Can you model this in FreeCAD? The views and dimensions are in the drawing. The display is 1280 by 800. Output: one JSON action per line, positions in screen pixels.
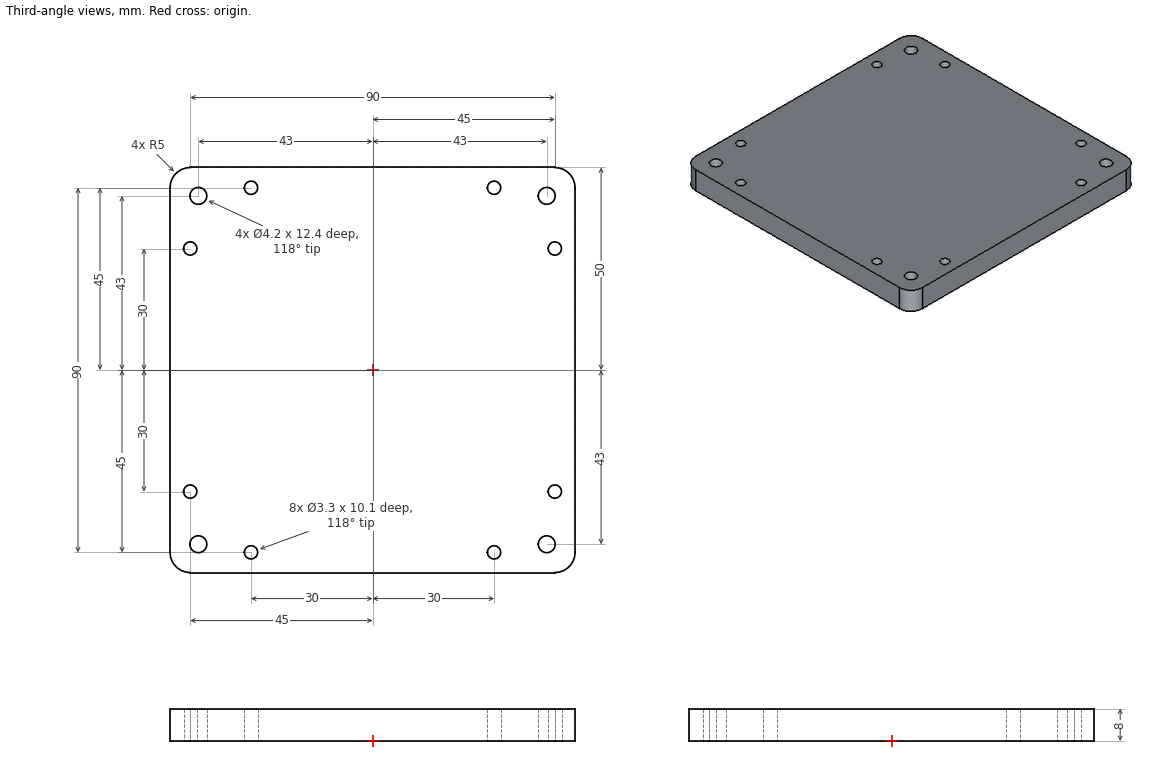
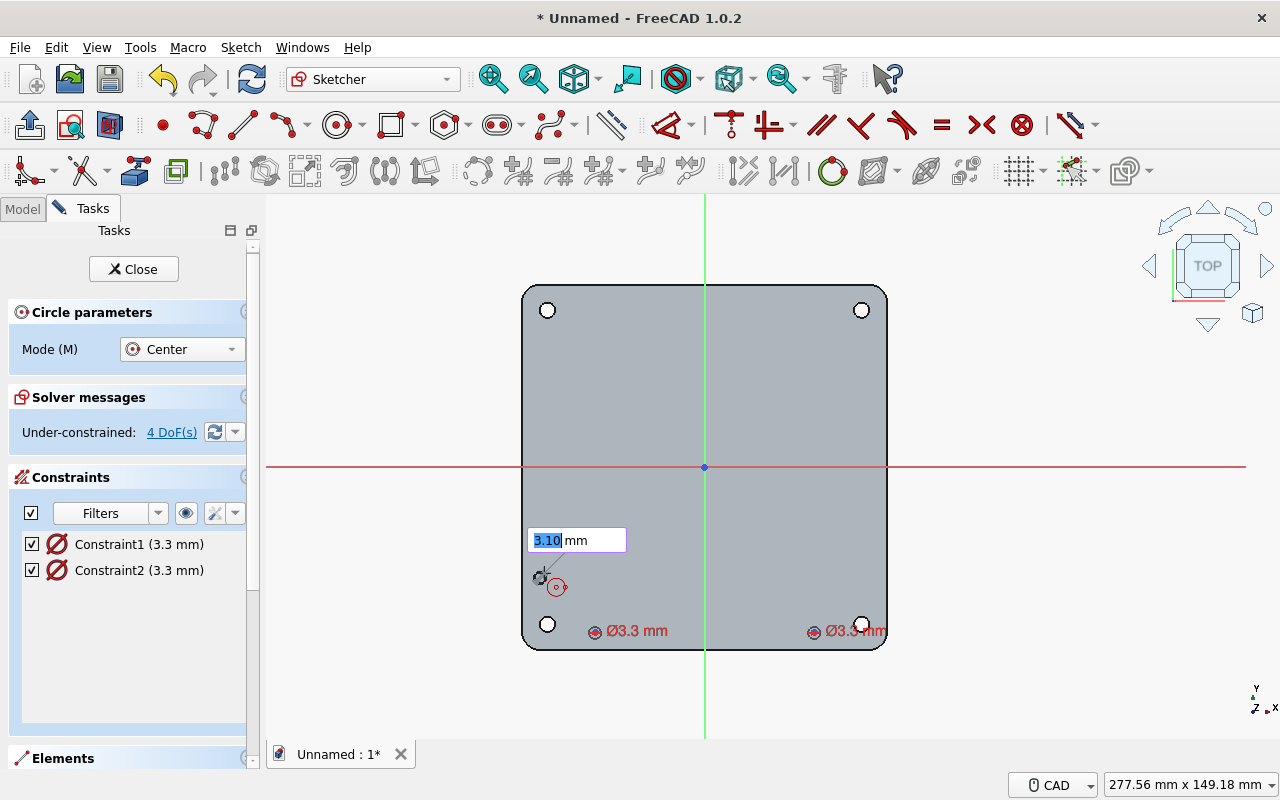
{"action": "type", "text": "3.3"}
{"action": "key", "text": "Return"}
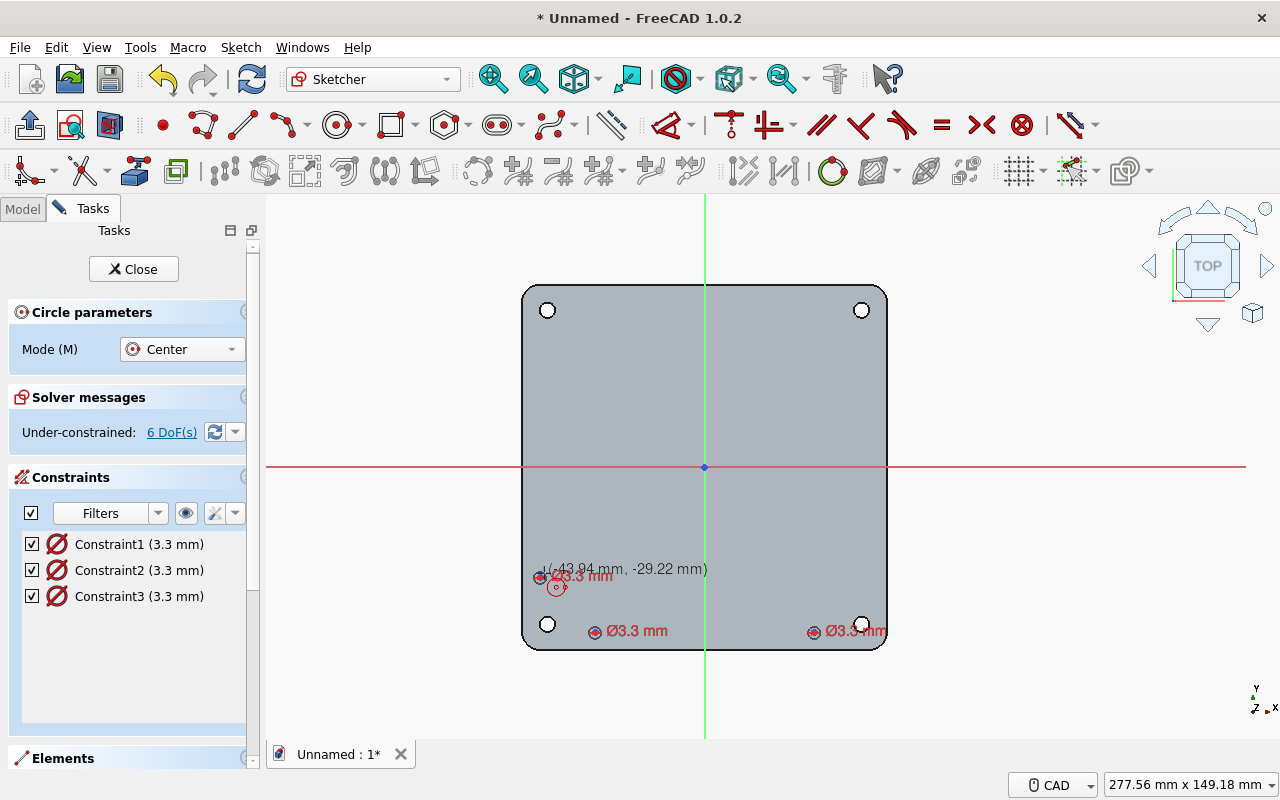
{"action": "scroll", "coordinate": [540, 358], "scroll_direction": "up", "scroll_amount": 7}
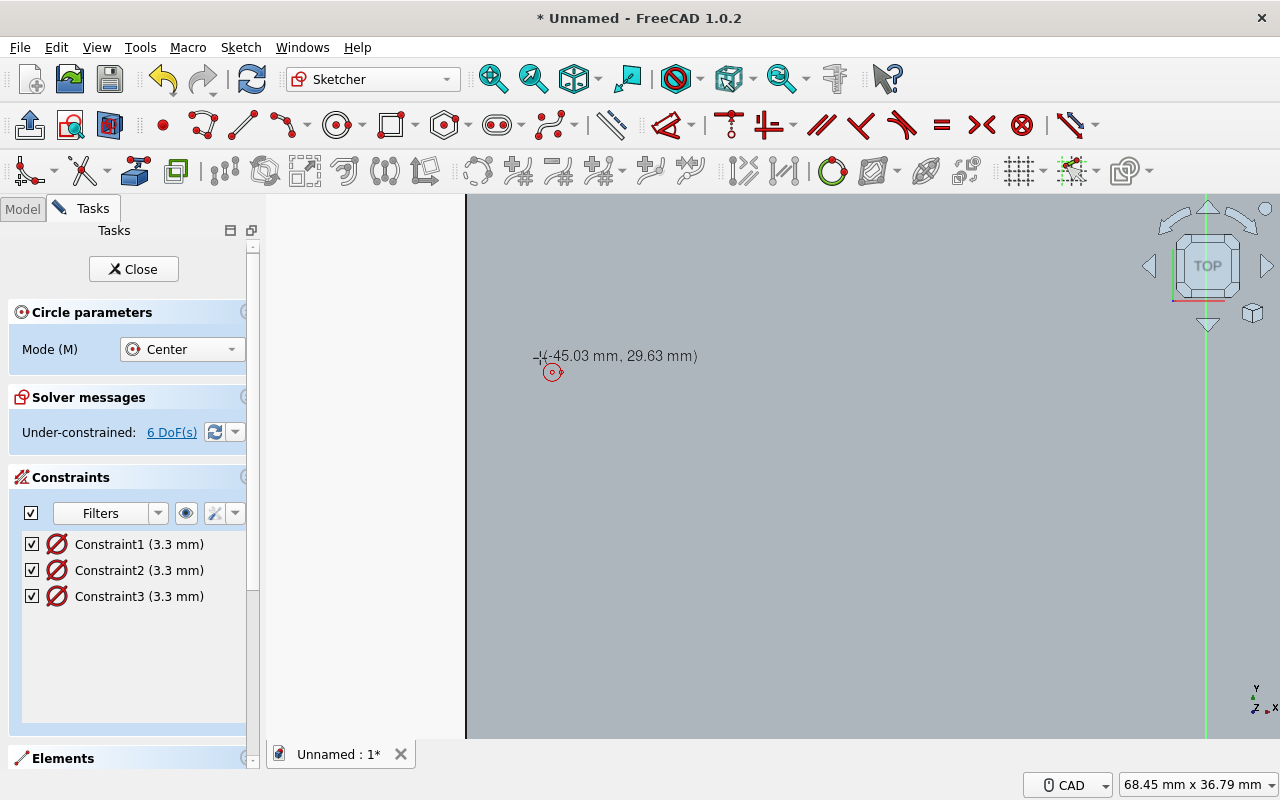
{"action": "scroll", "coordinate": [540, 357], "scroll_direction": "down", "scroll_amount": 7}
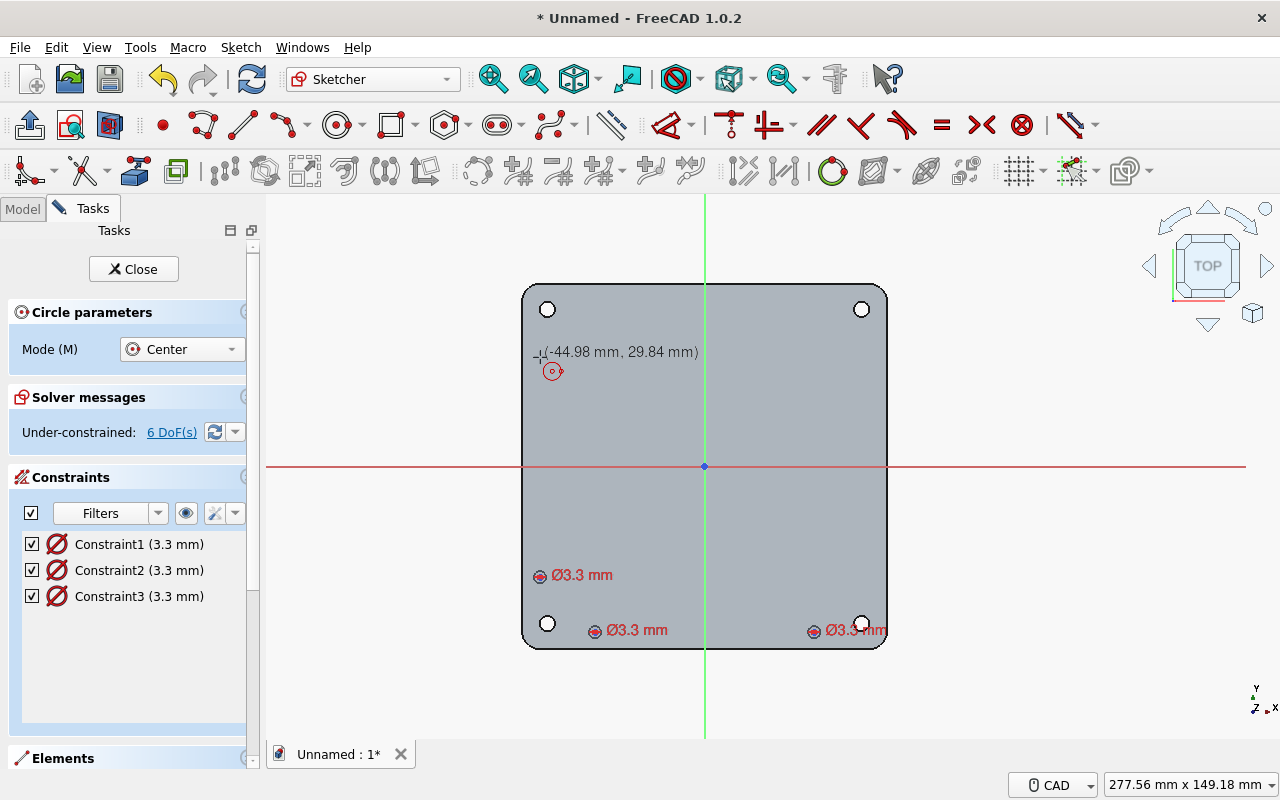
{"action": "left_click", "coordinate": [540, 357]}
{"action": "mouse_move", "coordinate": [544, 353]}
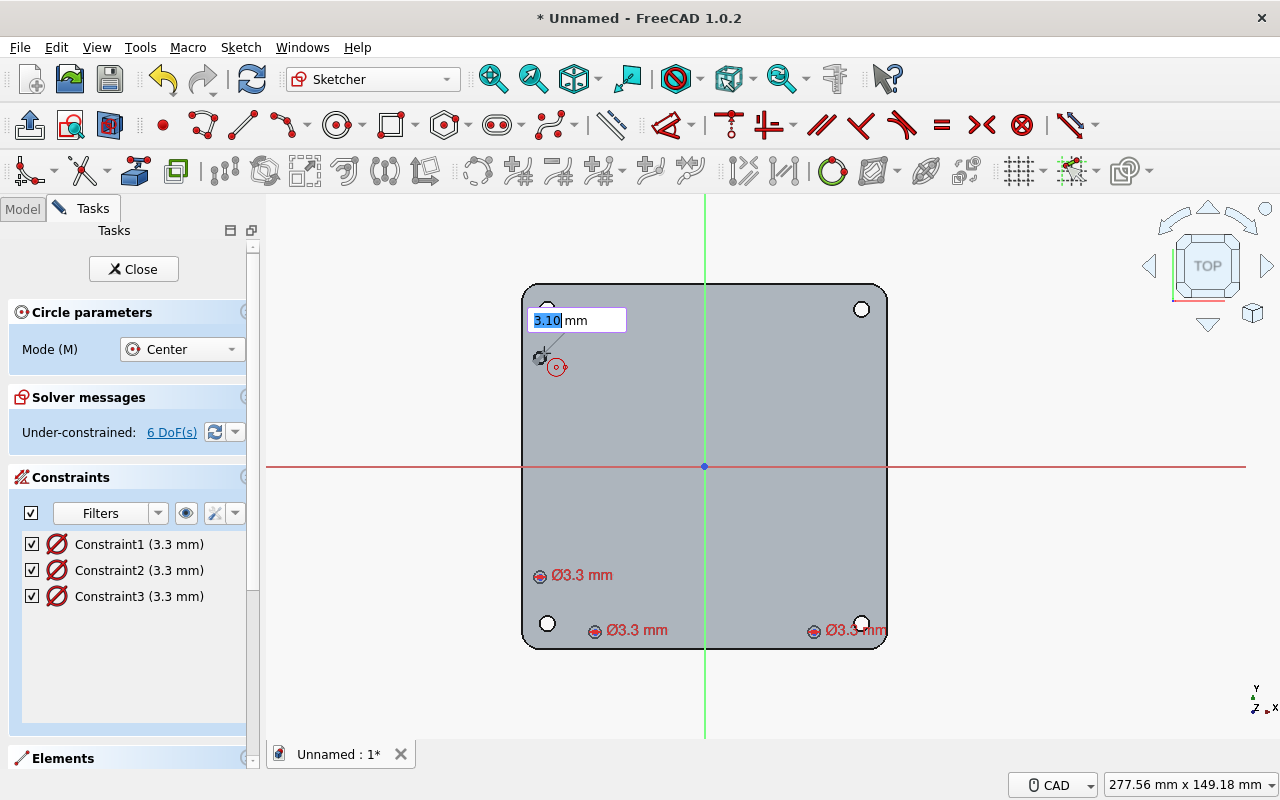
{"action": "type", "text": "3.3"}
{"action": "key", "text": "Return"}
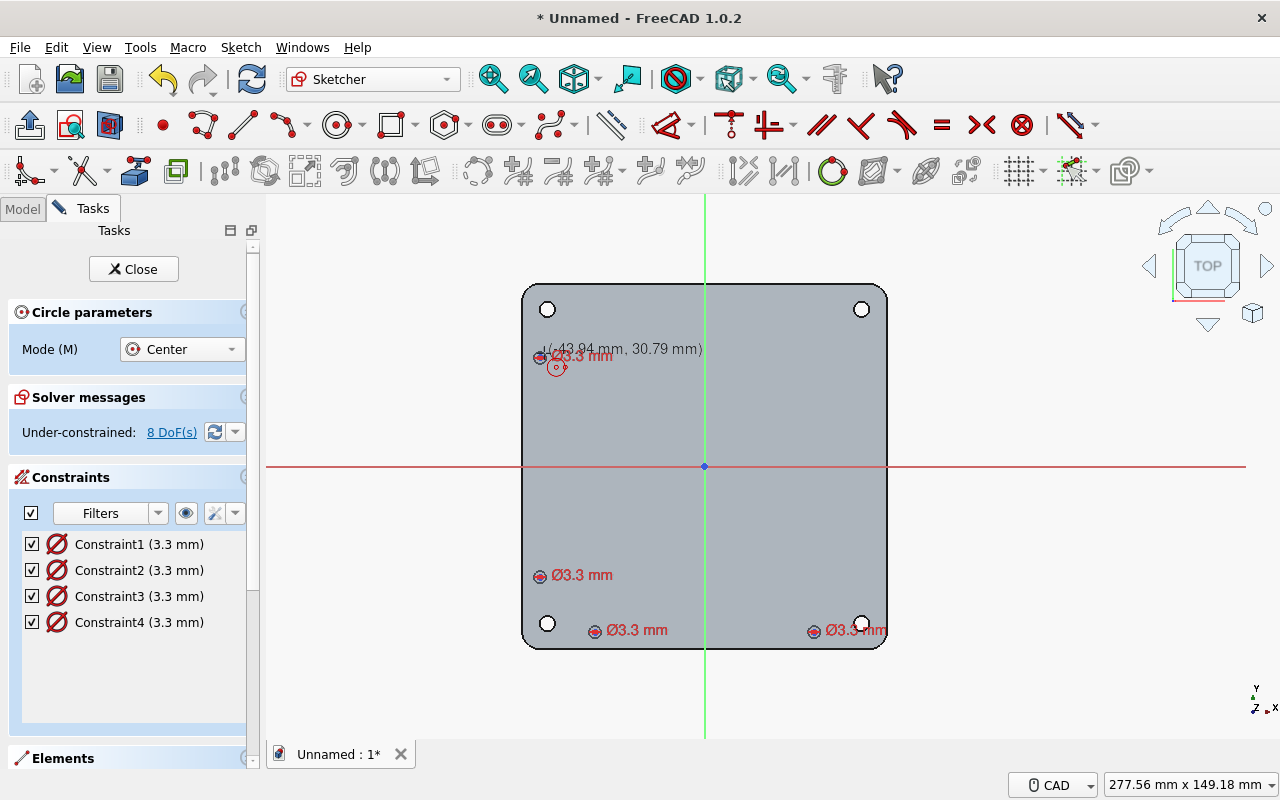
{"action": "scroll", "coordinate": [869, 357], "scroll_direction": "up", "scroll_amount": 7}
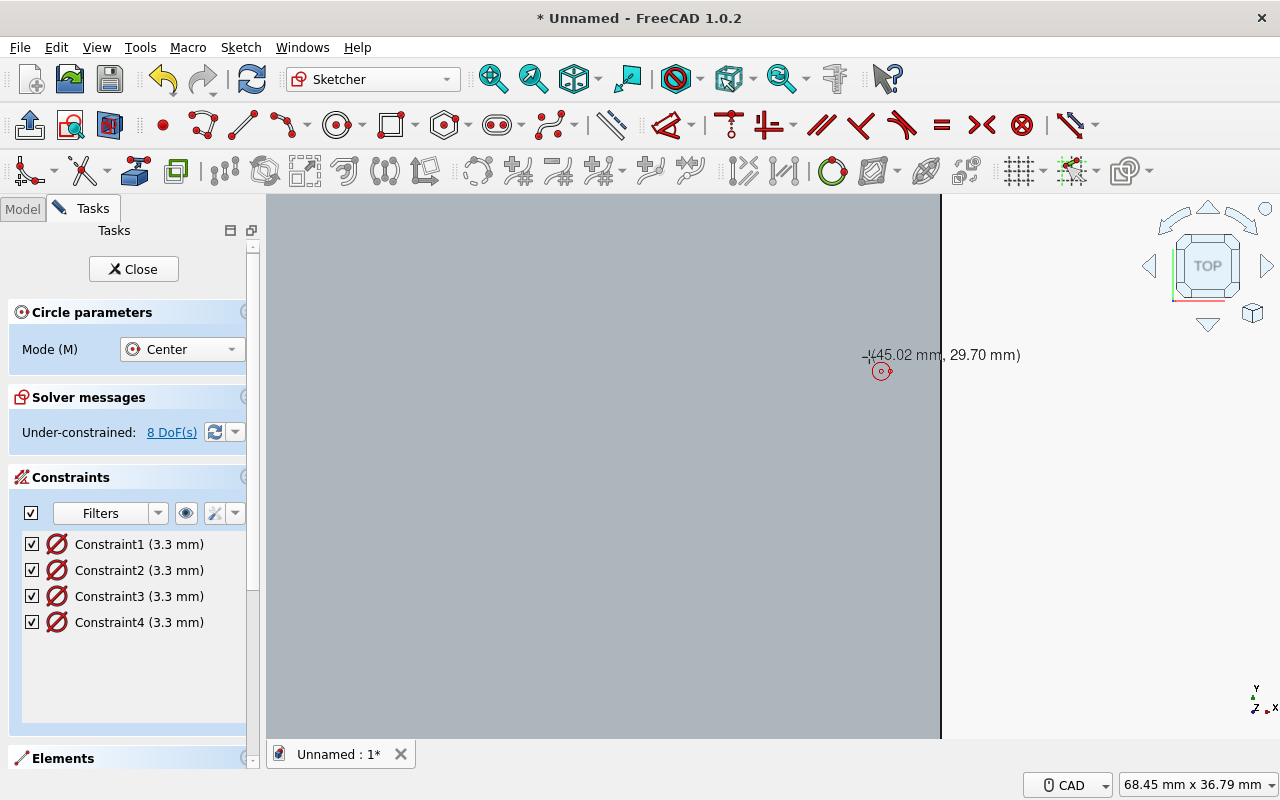
{"action": "scroll", "coordinate": [870, 357], "scroll_direction": "down", "scroll_amount": 7}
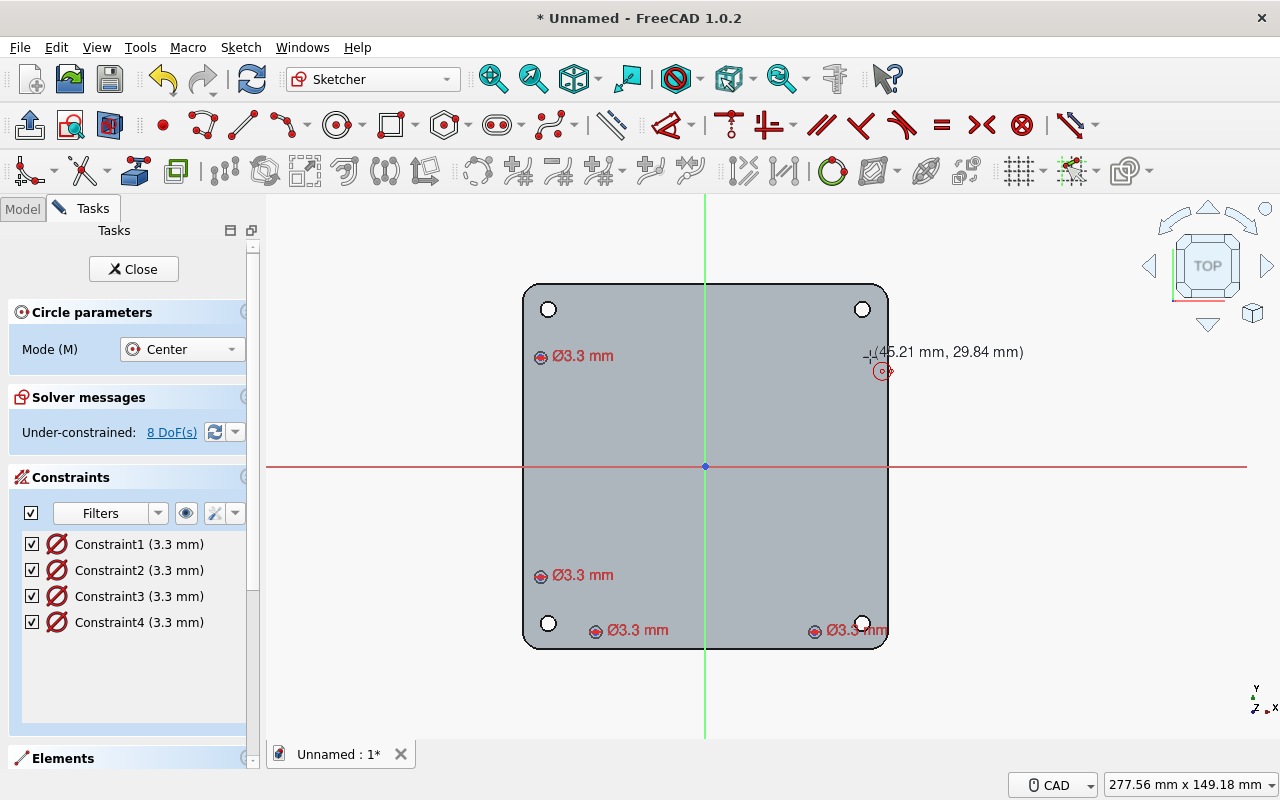
{"action": "left_click", "coordinate": [870, 357]}
{"action": "mouse_move", "coordinate": [874, 353]}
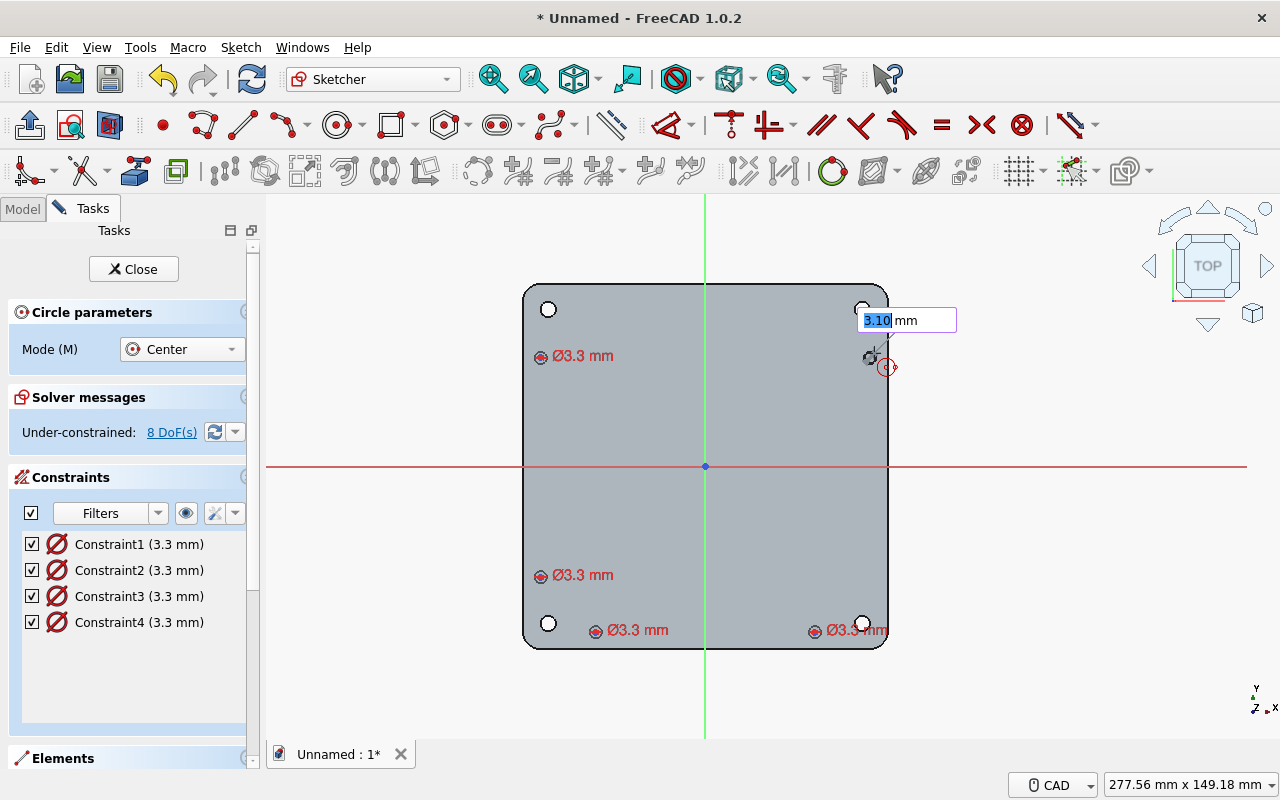
{"action": "type", "text": "3.3"}
{"action": "key", "text": "Return"}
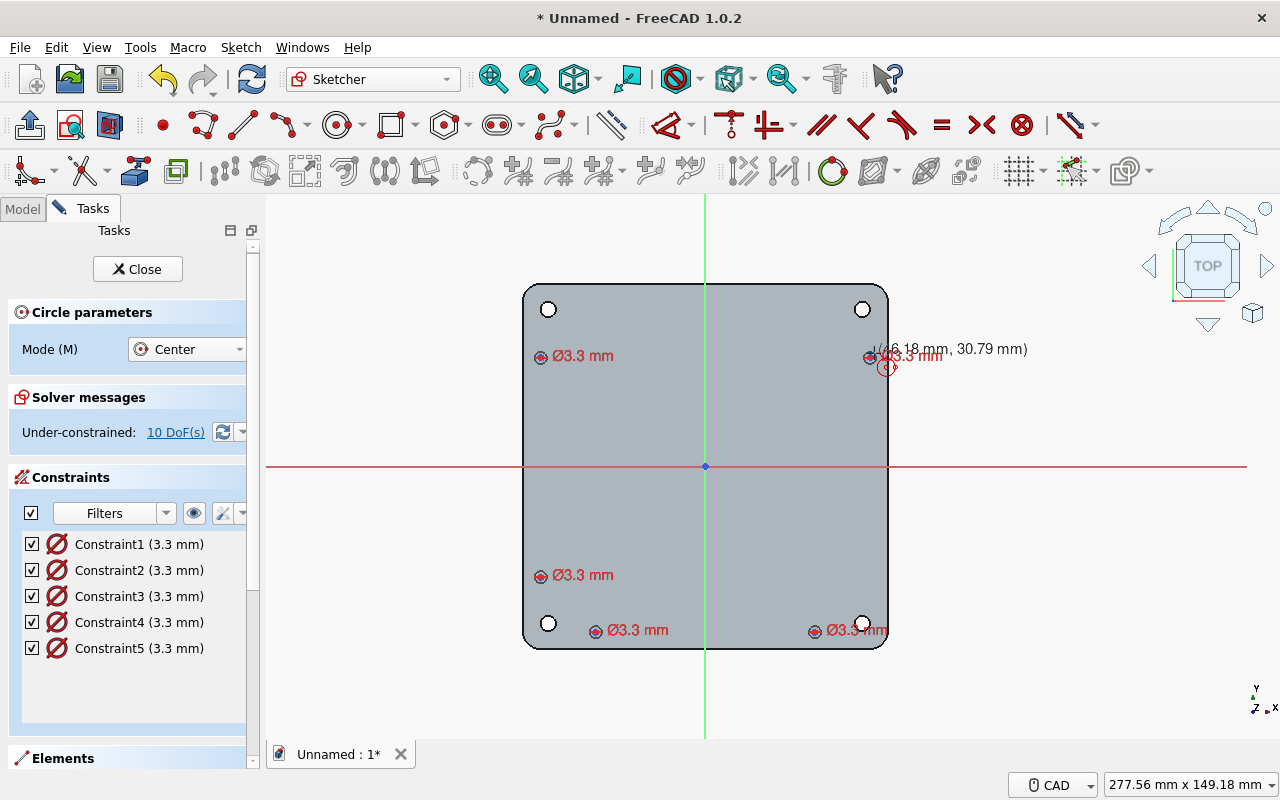
{"action": "scroll", "coordinate": [870, 576], "scroll_direction": "up", "scroll_amount": 7}